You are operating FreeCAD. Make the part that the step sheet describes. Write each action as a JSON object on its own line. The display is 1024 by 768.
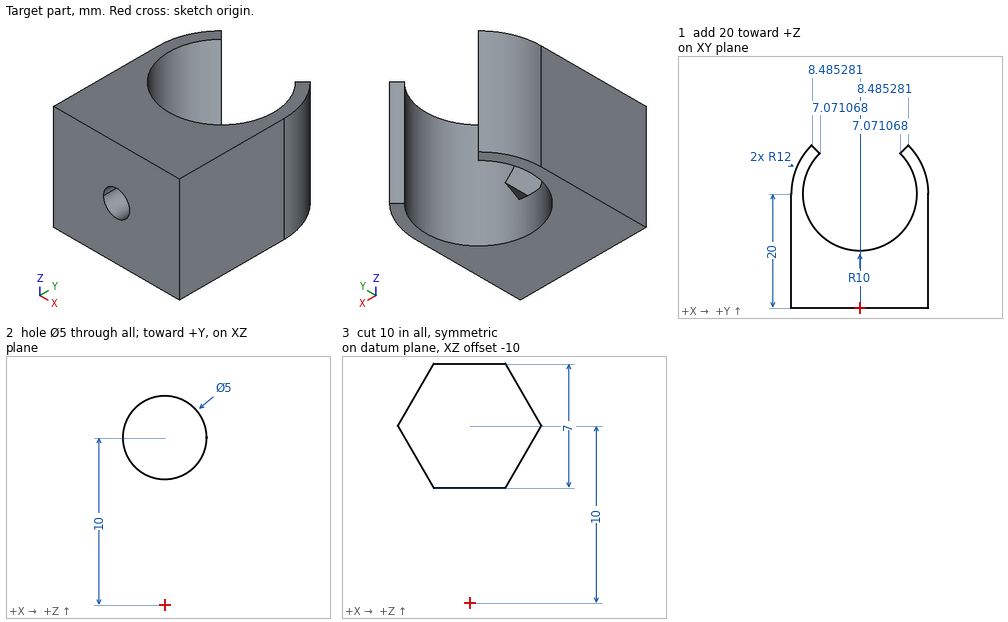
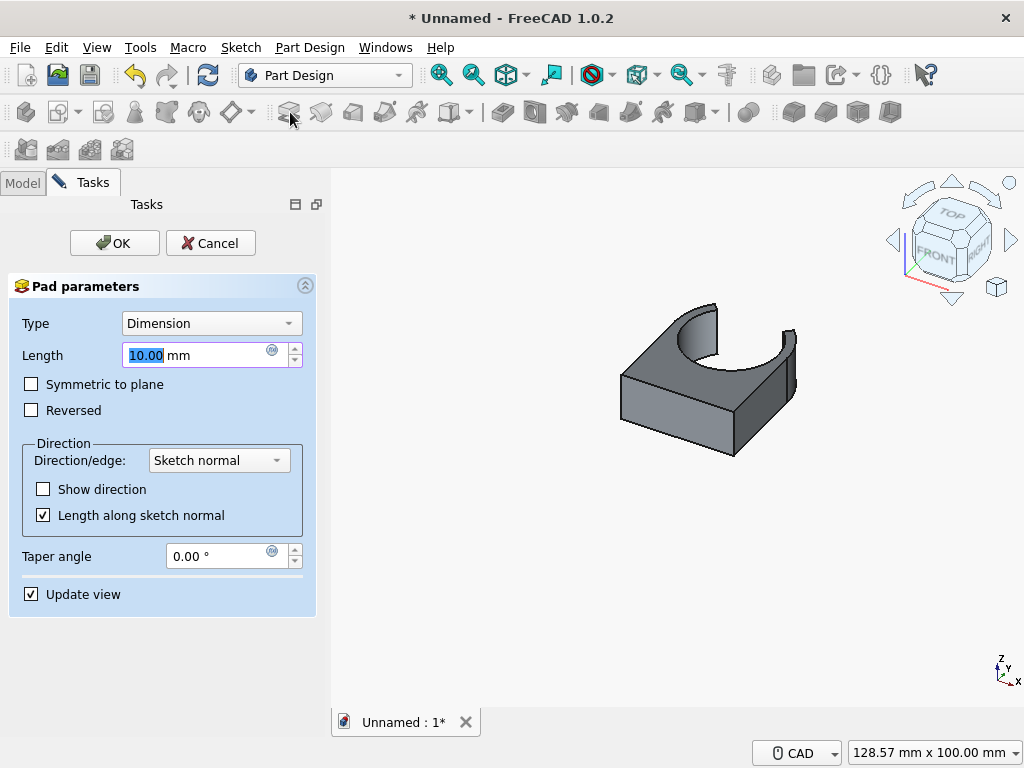
{"action": "type", "text": "20"}
{"action": "key", "text": "Tab"}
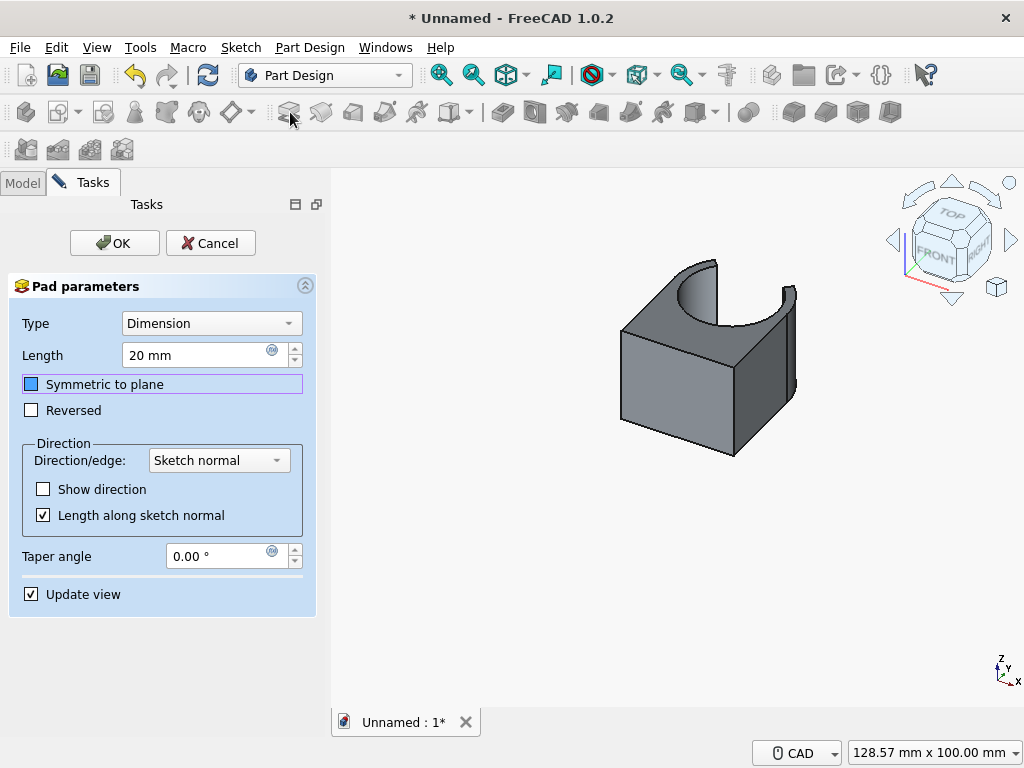
{"action": "left_click", "coordinate": [115, 243]}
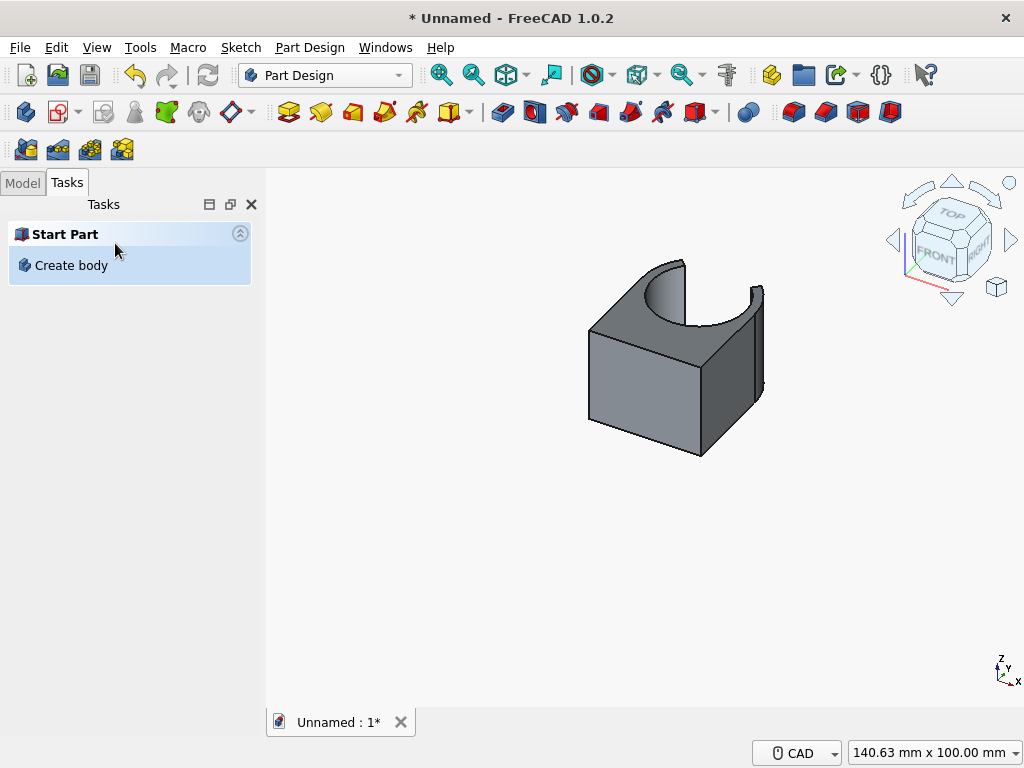
{"action": "left_click", "coordinate": [442, 76]}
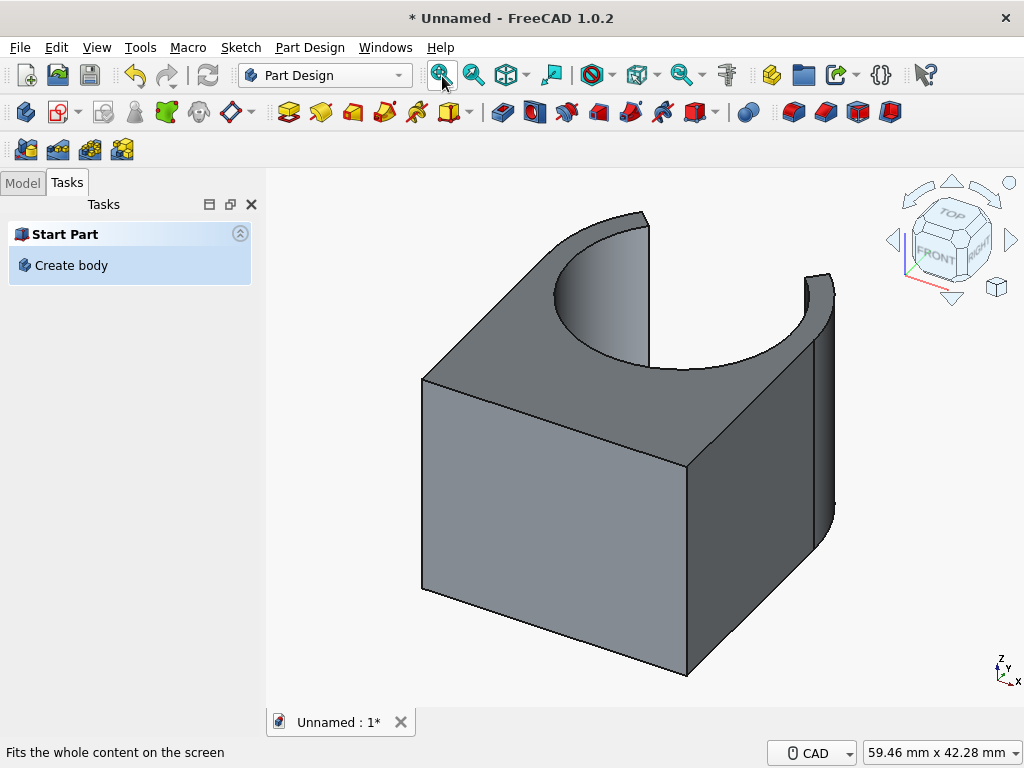
{"action": "left_click", "coordinate": [58, 112]}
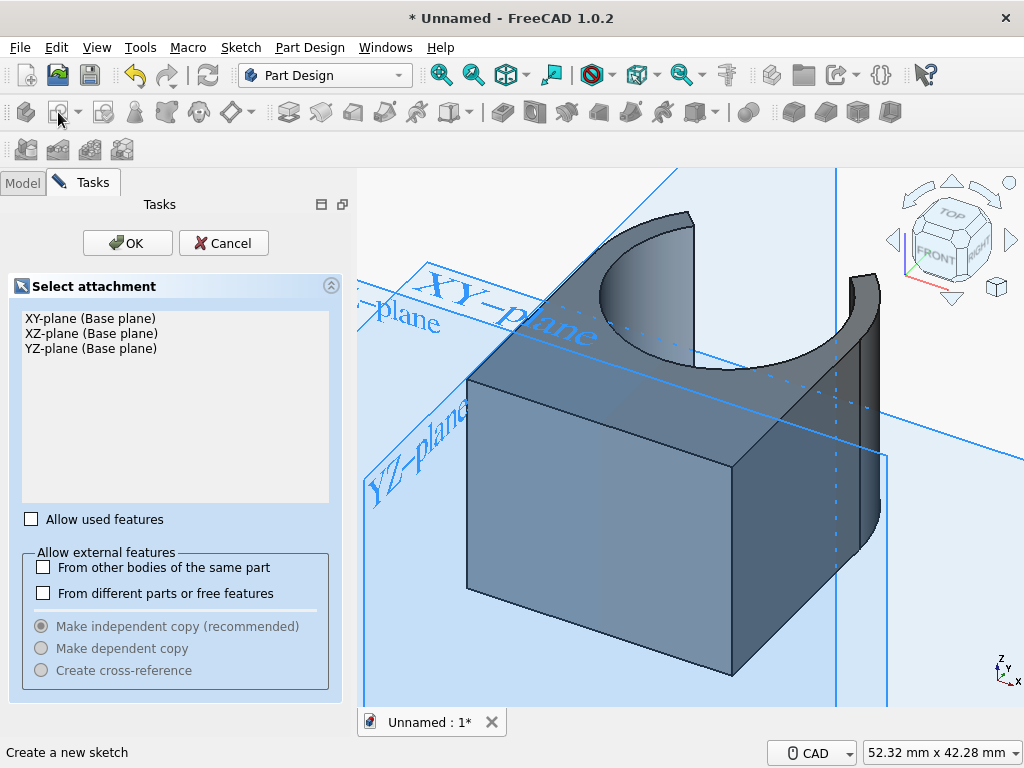
{"action": "left_click", "coordinate": [82, 334]}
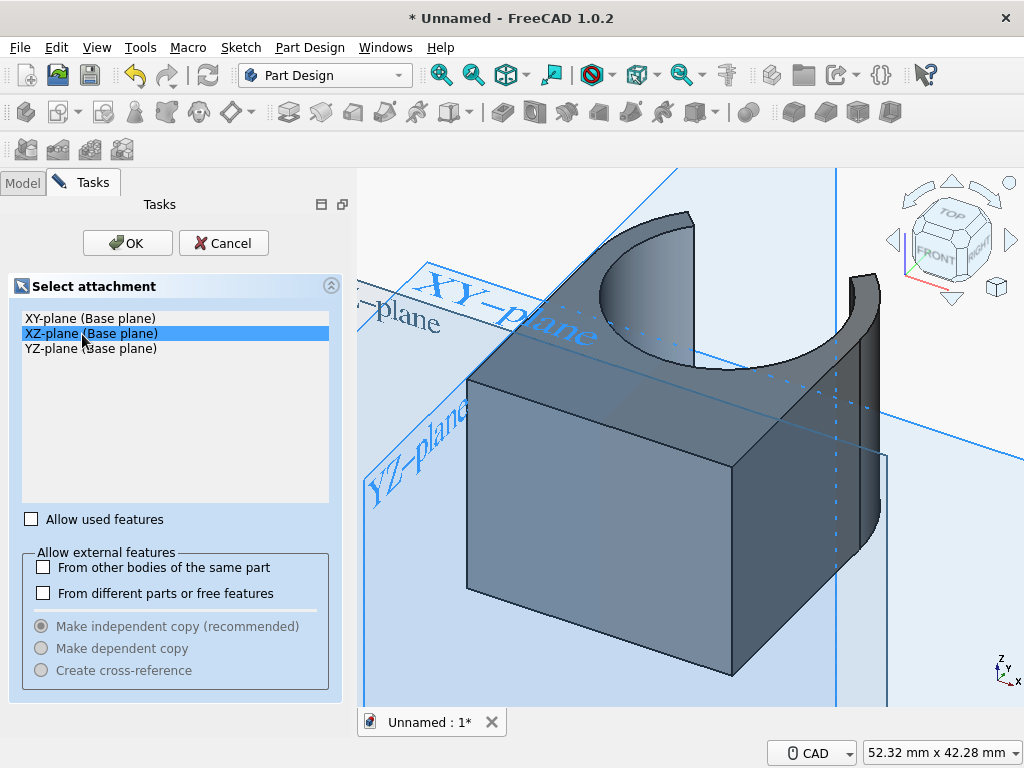
{"action": "left_click", "coordinate": [128, 243]}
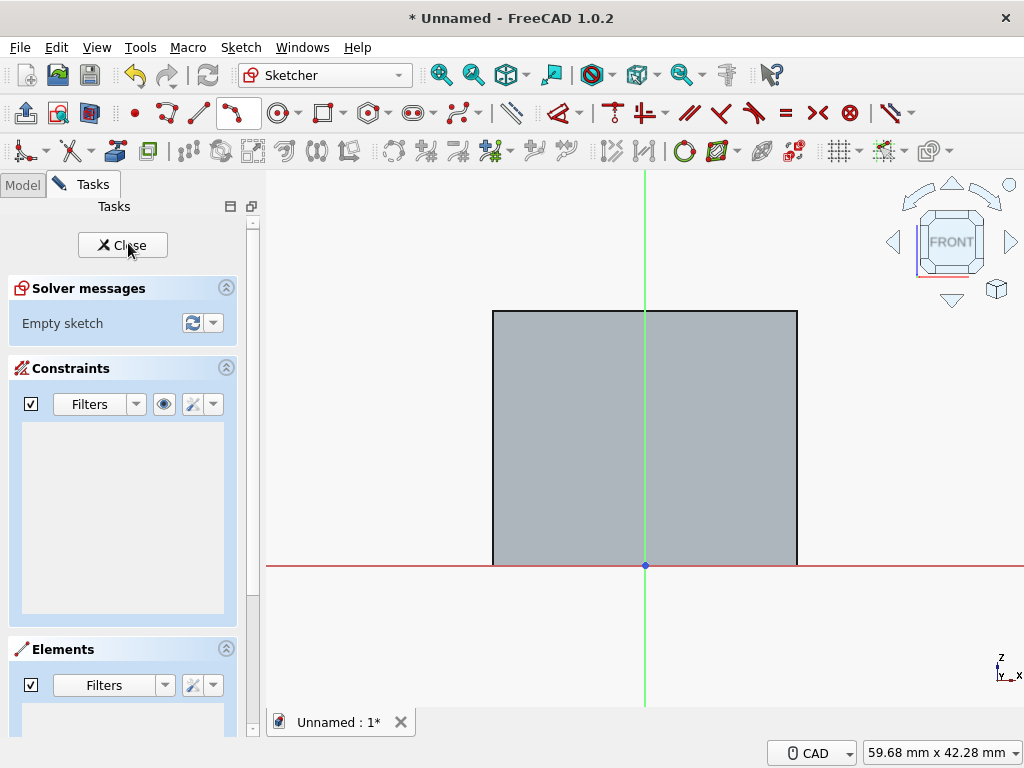
{"action": "scroll", "coordinate": [662, 438], "scroll_direction": "up", "scroll_amount": 8}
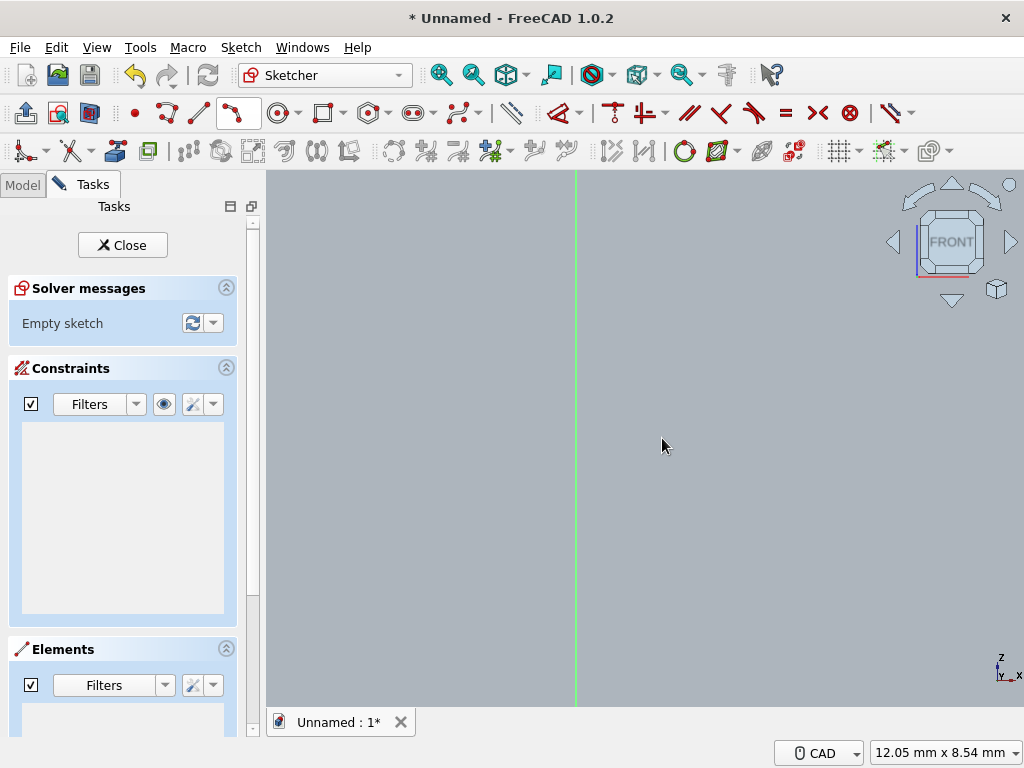
{"action": "key", "text": "g c"}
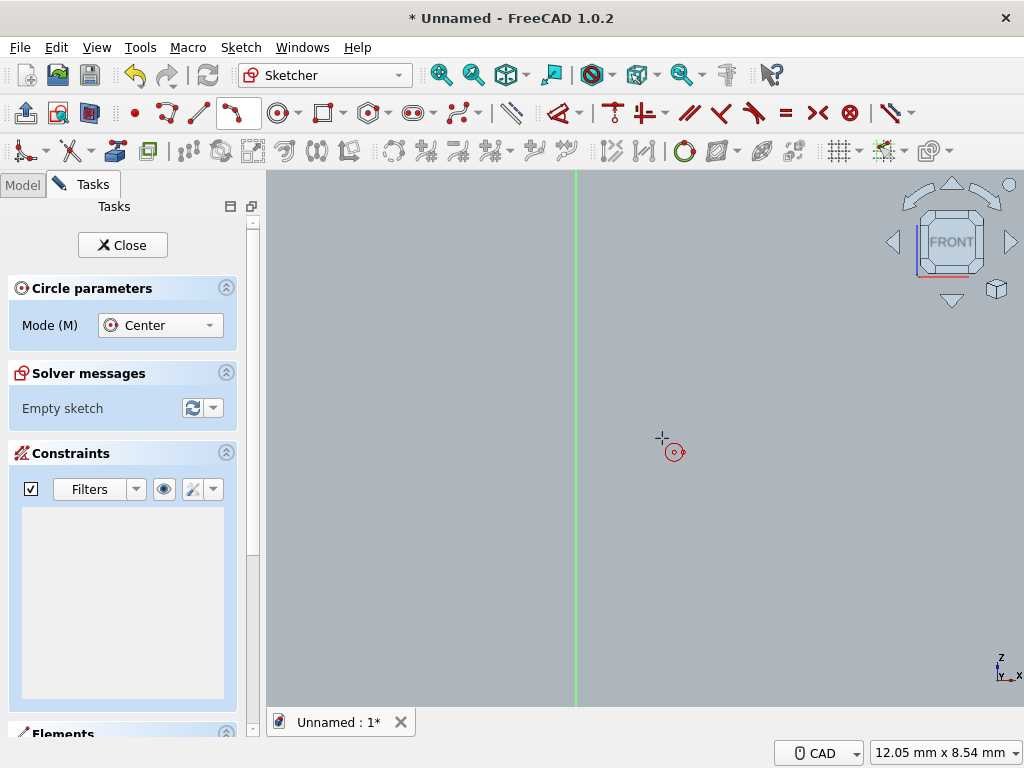
{"action": "left_click", "coordinate": [576, 438]}
{"action": "mouse_move", "coordinate": [687, 327]}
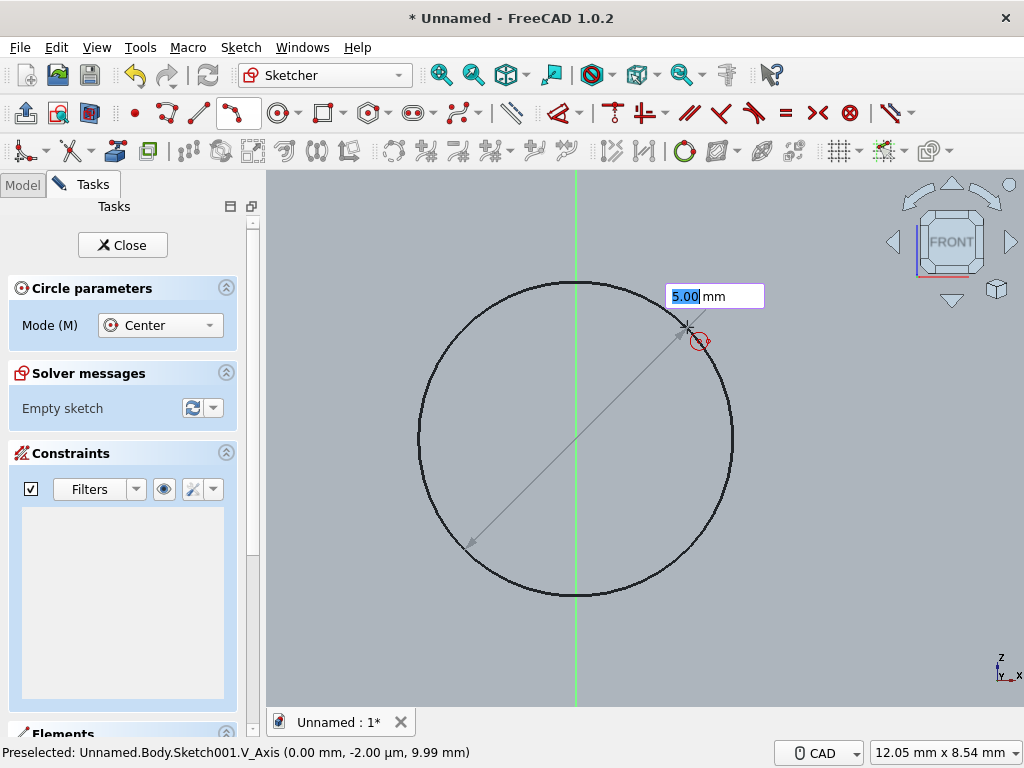
{"action": "type", "text": "5"}
{"action": "key", "text": "Return"}
{"action": "key", "text": "Escape"}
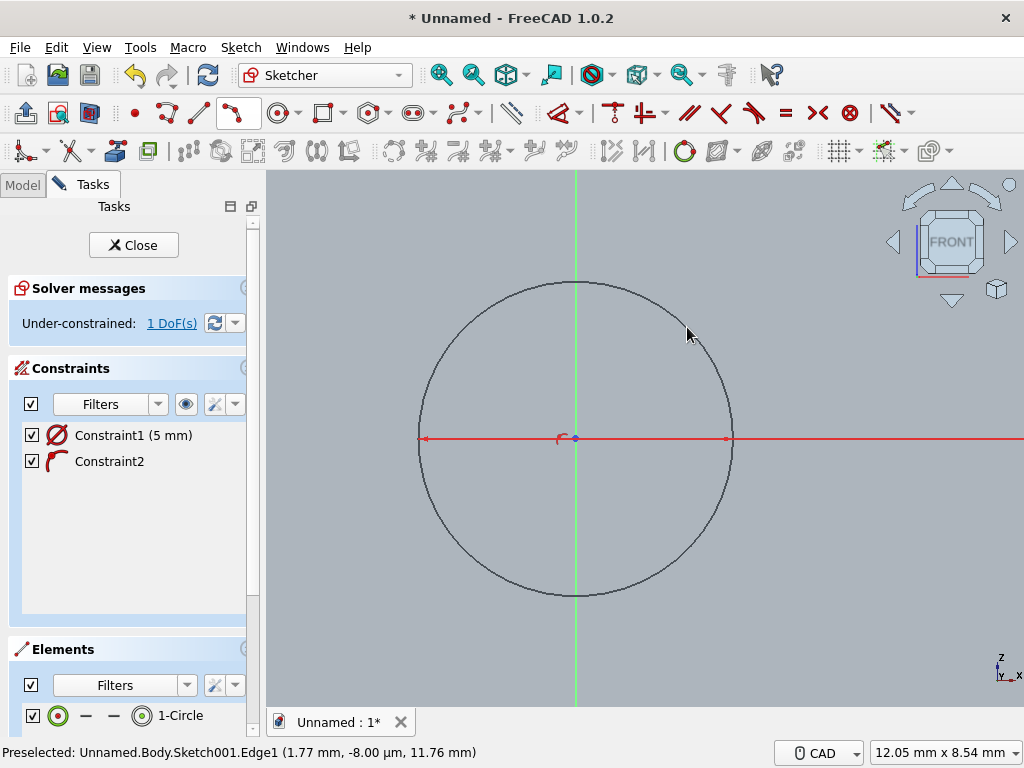
{"action": "left_click", "coordinate": [558, 114]}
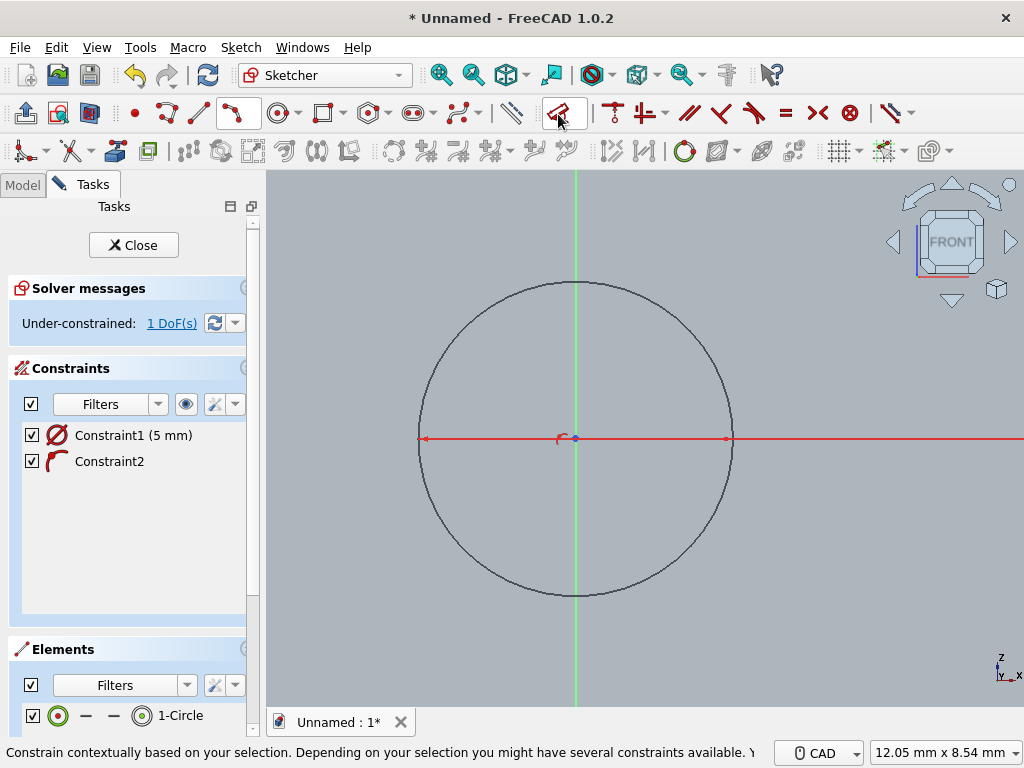
{"action": "left_click", "coordinate": [576, 439]}
{"action": "left_click", "coordinate": [610, 559]}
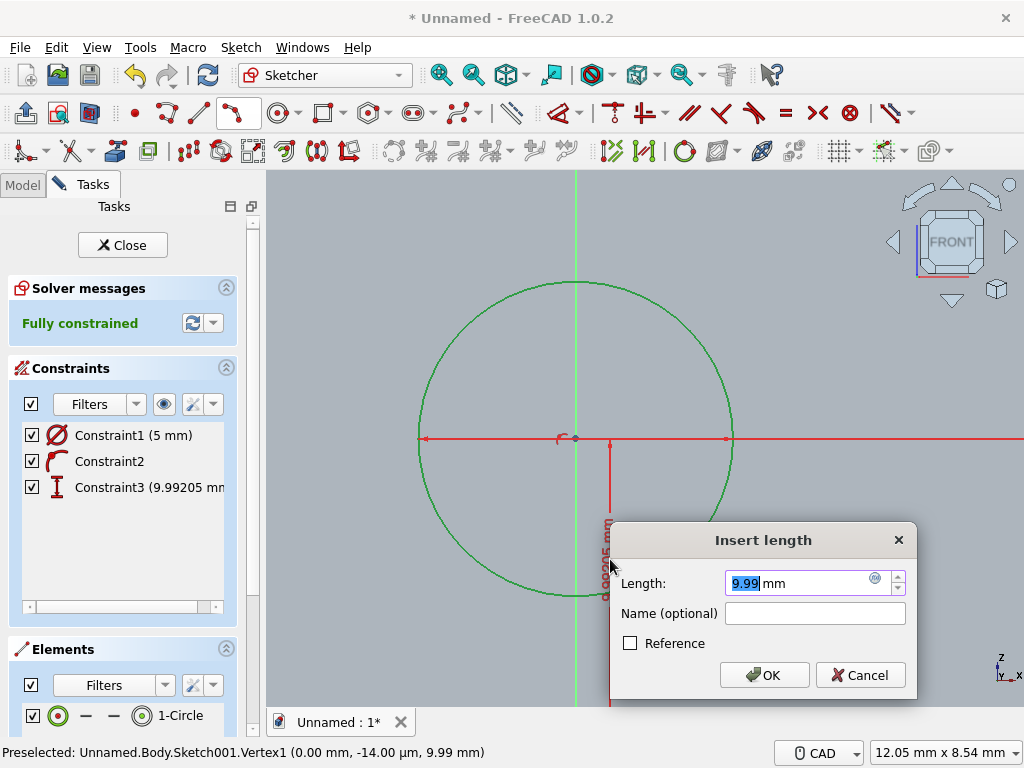
{"action": "type", "text": "10"}
{"action": "key", "text": "Return"}
{"action": "key", "text": "Escape"}